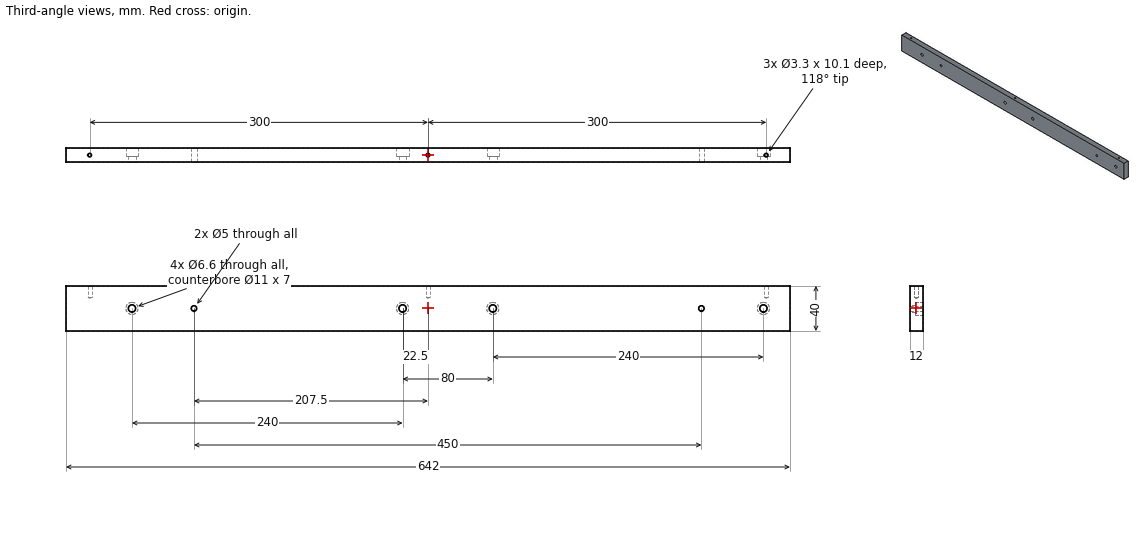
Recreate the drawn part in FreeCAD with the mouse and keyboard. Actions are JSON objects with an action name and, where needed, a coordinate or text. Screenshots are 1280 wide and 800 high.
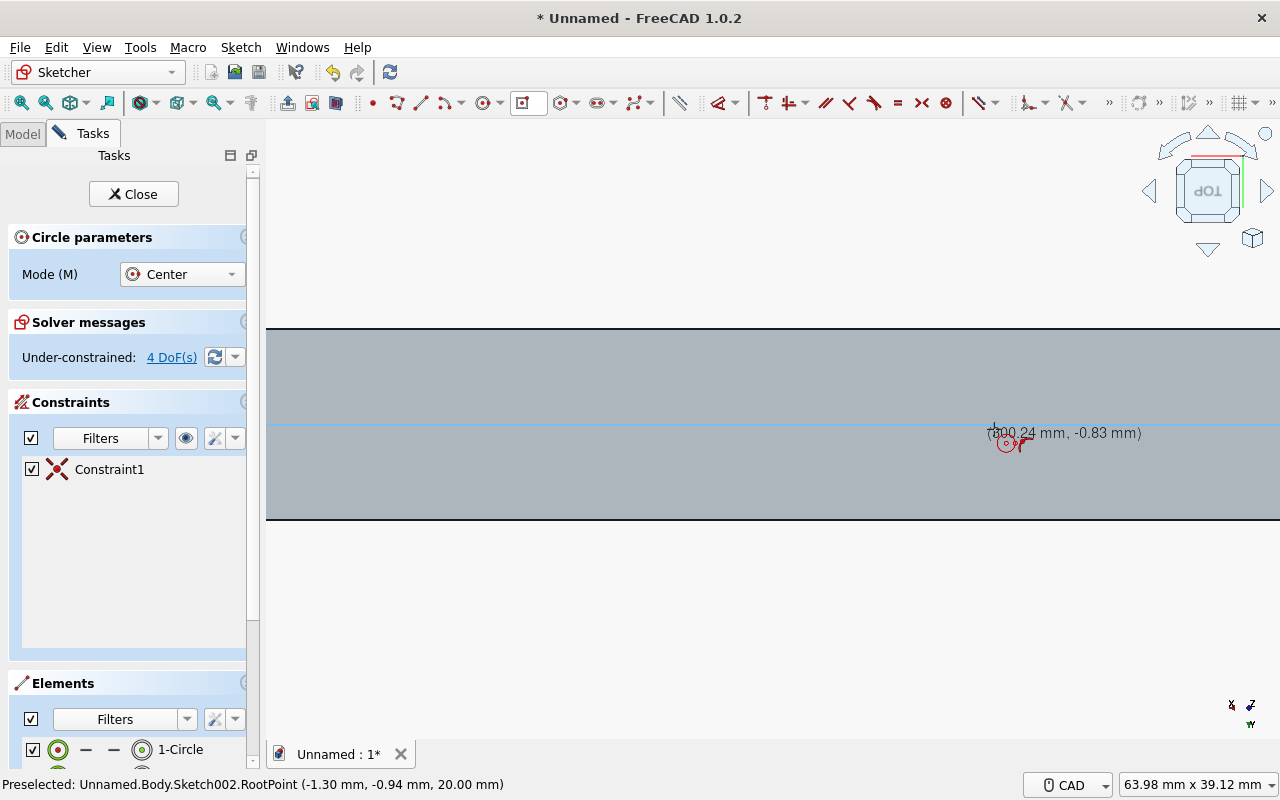
{"action": "scroll", "coordinate": [995, 429], "scroll_direction": "down", "scroll_amount": 14}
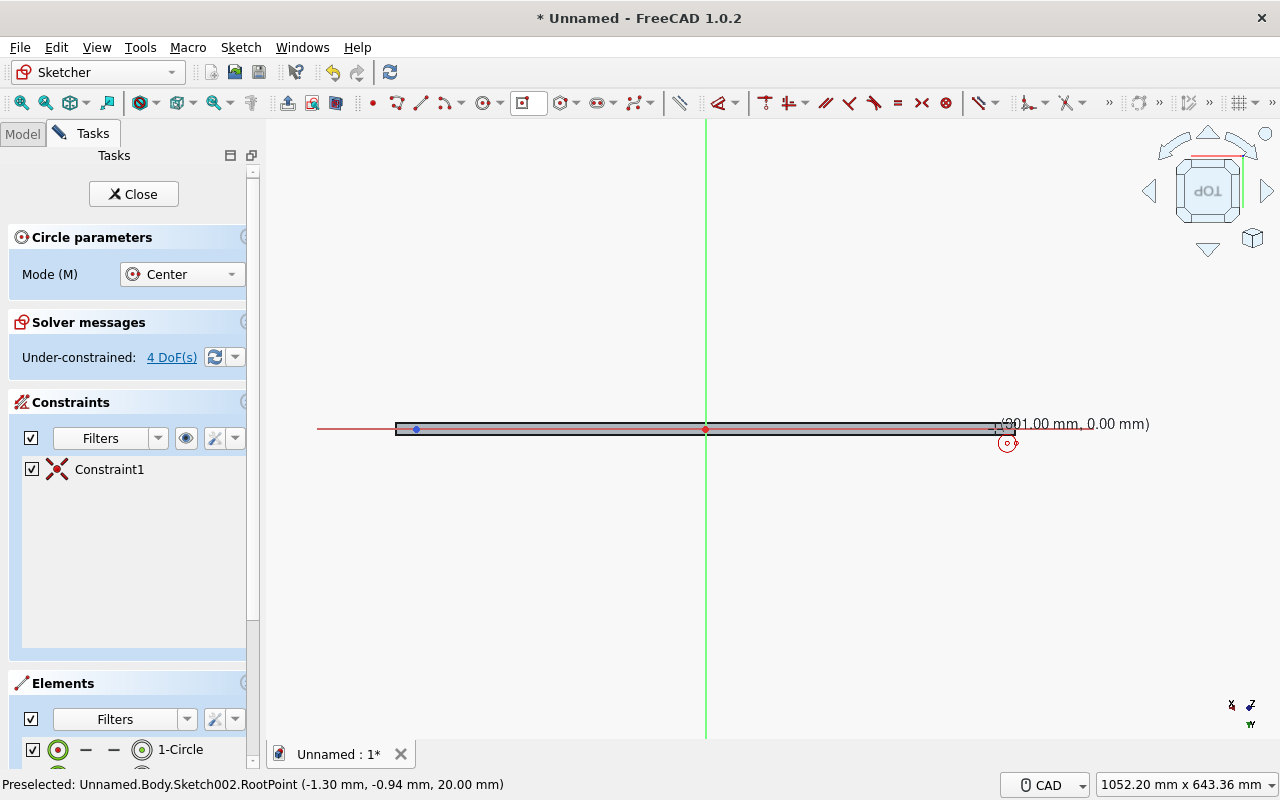
{"action": "left_click", "coordinate": [995, 429]}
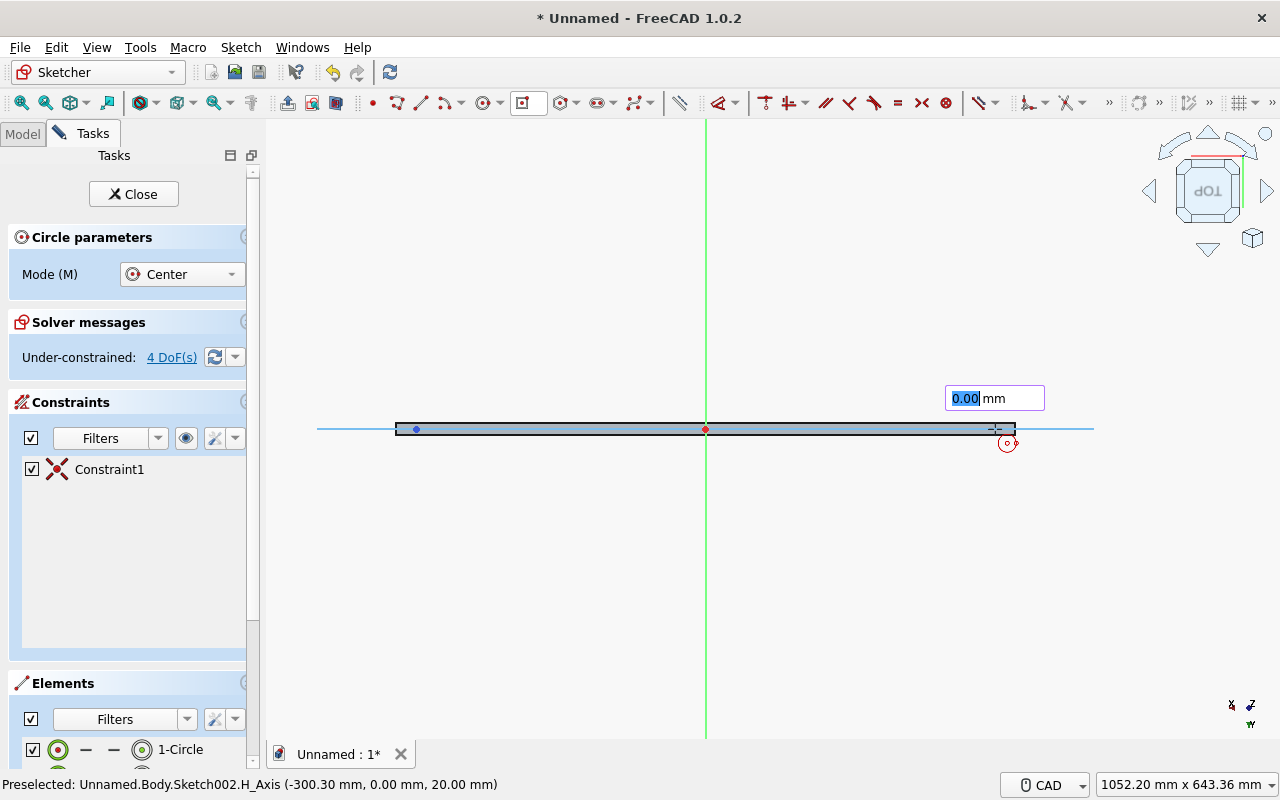
{"action": "scroll", "coordinate": [994, 431], "scroll_direction": "up", "scroll_amount": 12}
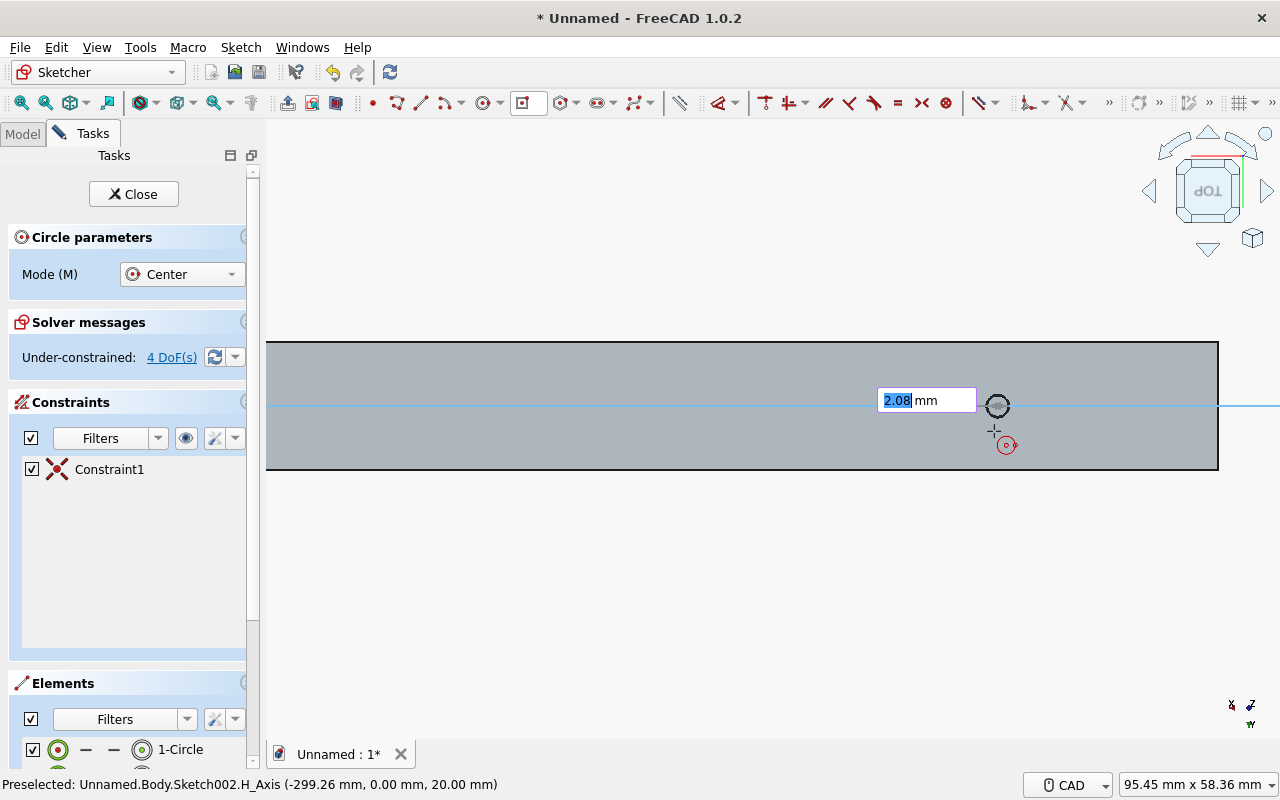
{"action": "left_click", "coordinate": [989, 423]}
{"action": "key", "text": "Escape"}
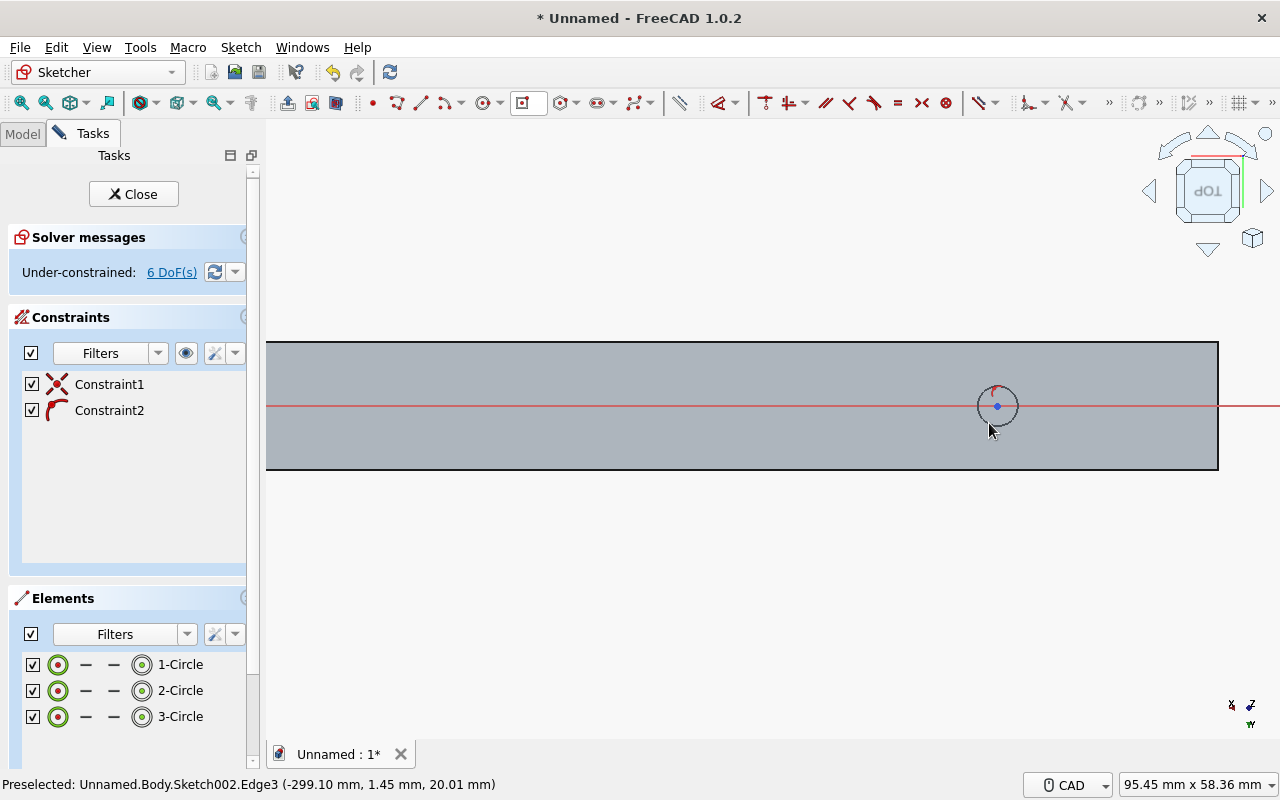
{"action": "scroll", "coordinate": [994, 431], "scroll_direction": "down", "scroll_amount": 12}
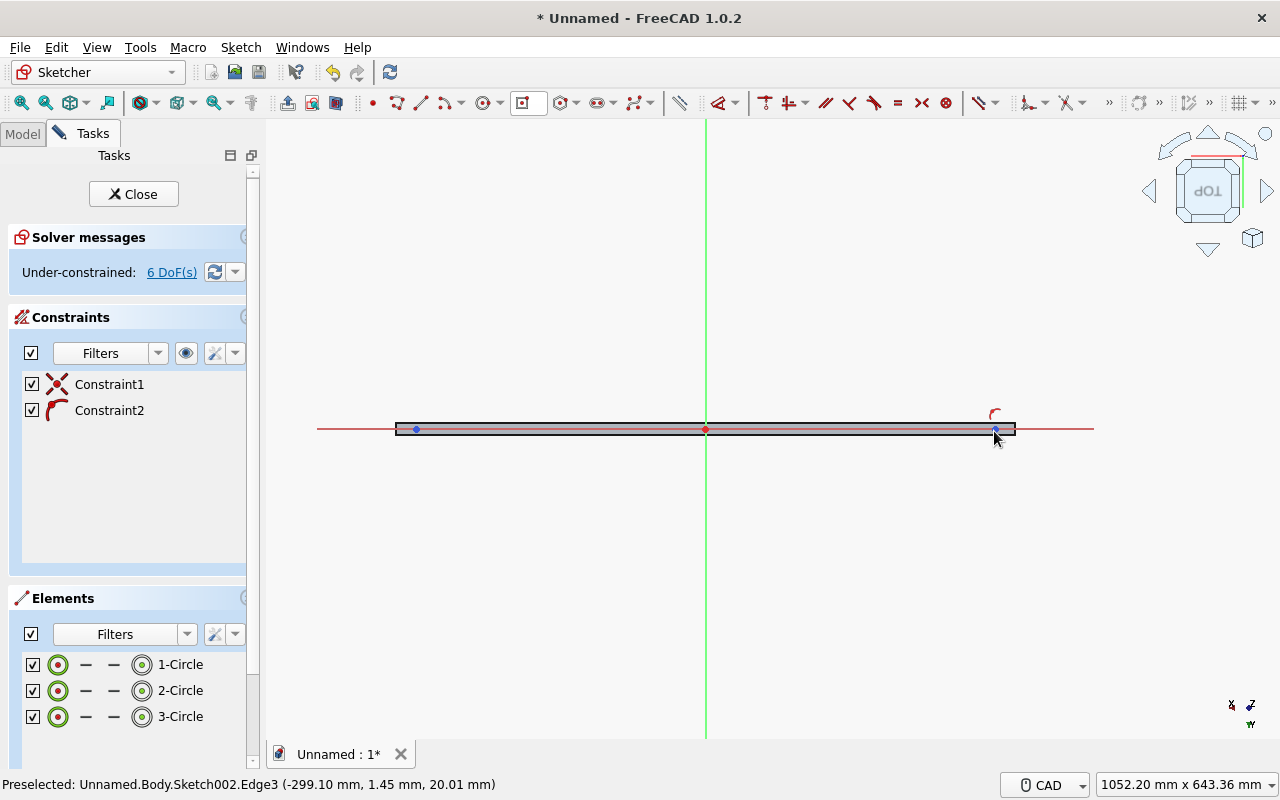
{"action": "scroll", "coordinate": [418, 429], "scroll_direction": "up", "scroll_amount": 12}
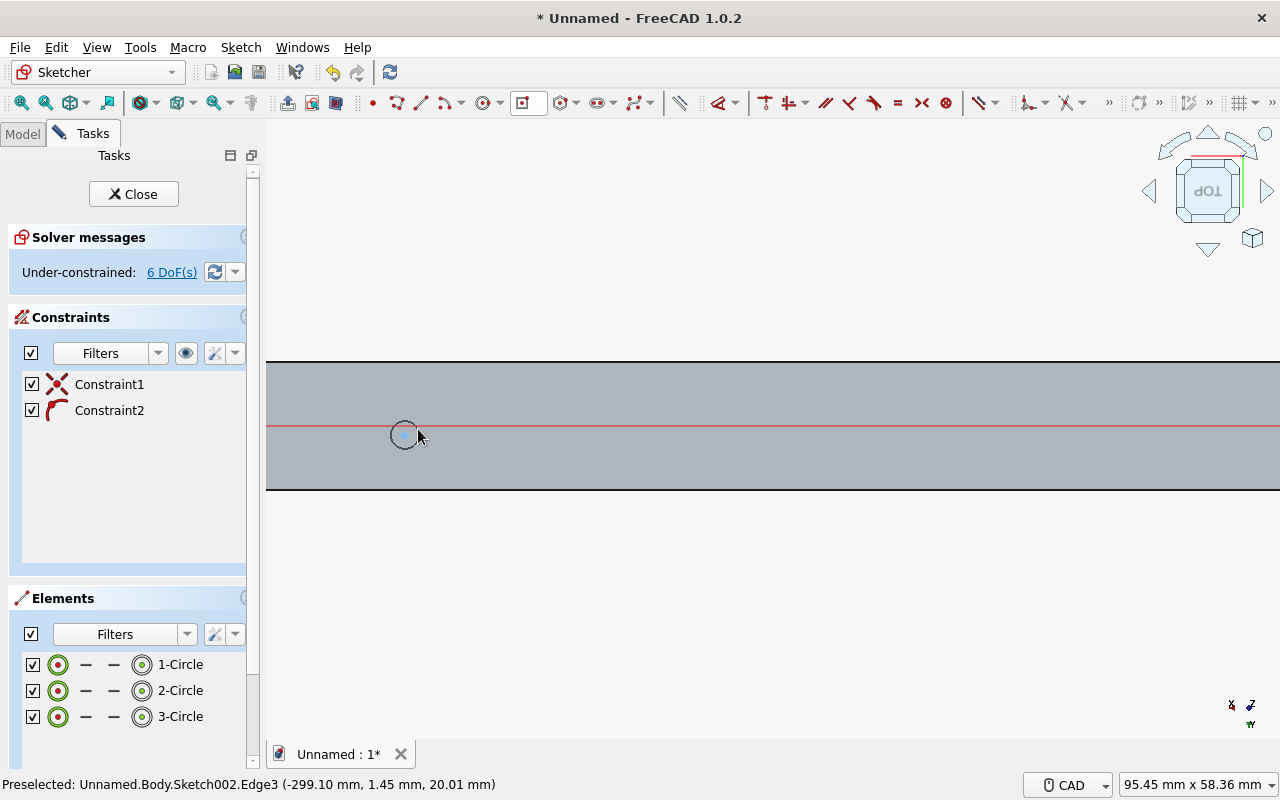
{"action": "left_click", "coordinate": [415, 425]}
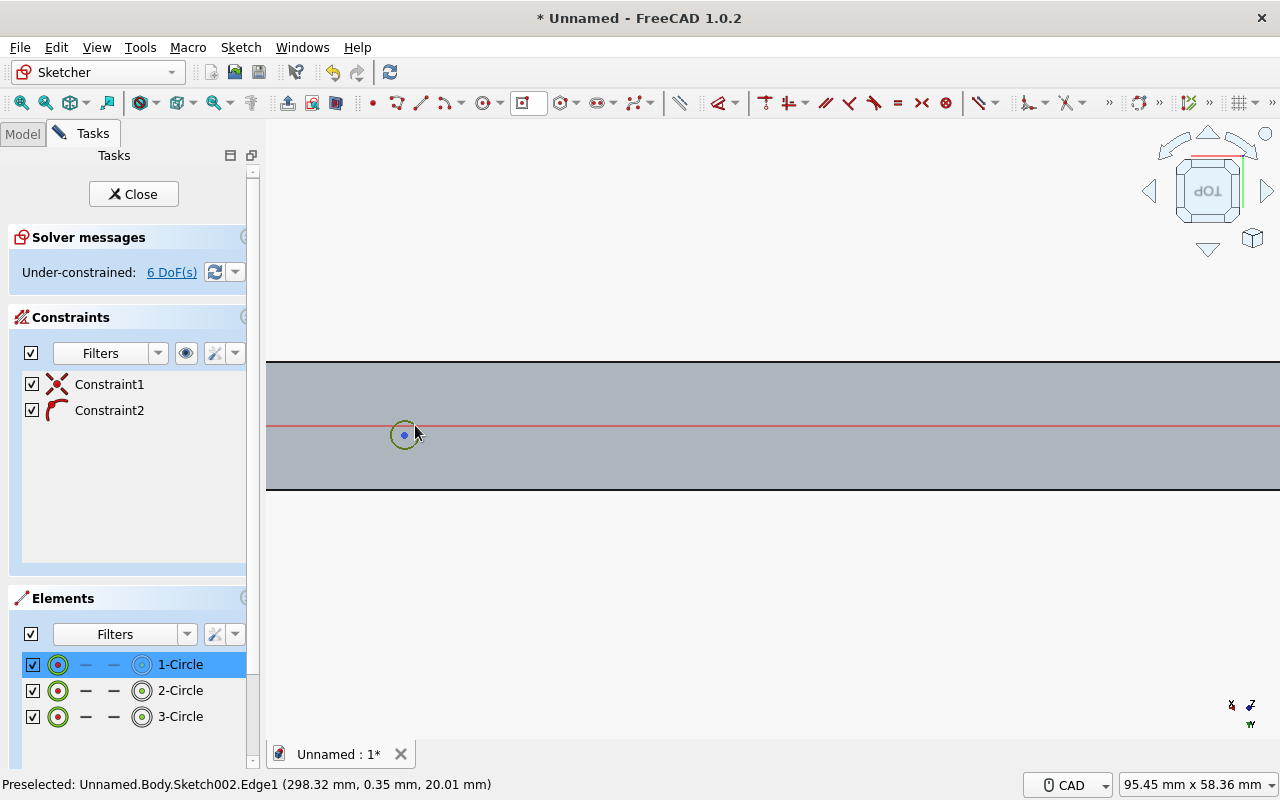
{"action": "scroll", "coordinate": [417, 429], "scroll_direction": "down", "scroll_amount": 12}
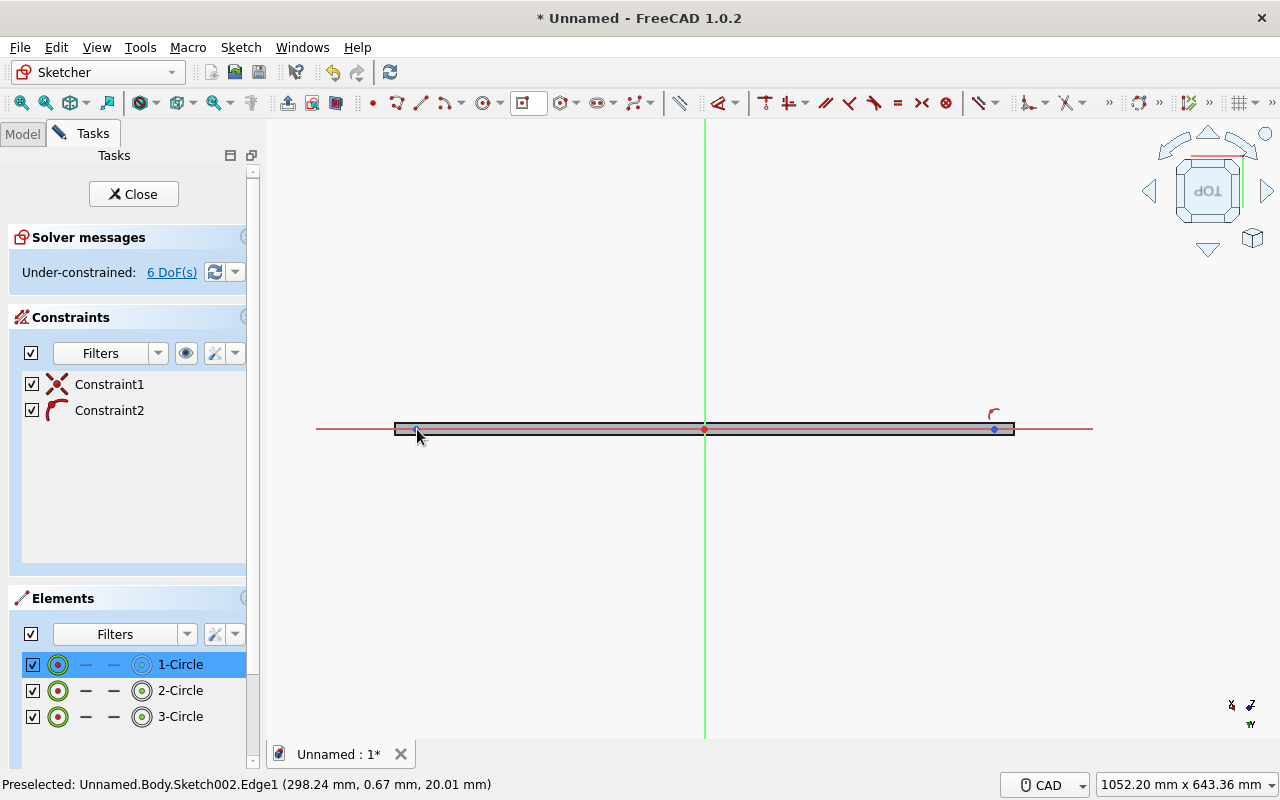
{"action": "scroll", "coordinate": [706, 428], "scroll_direction": "up", "scroll_amount": 13}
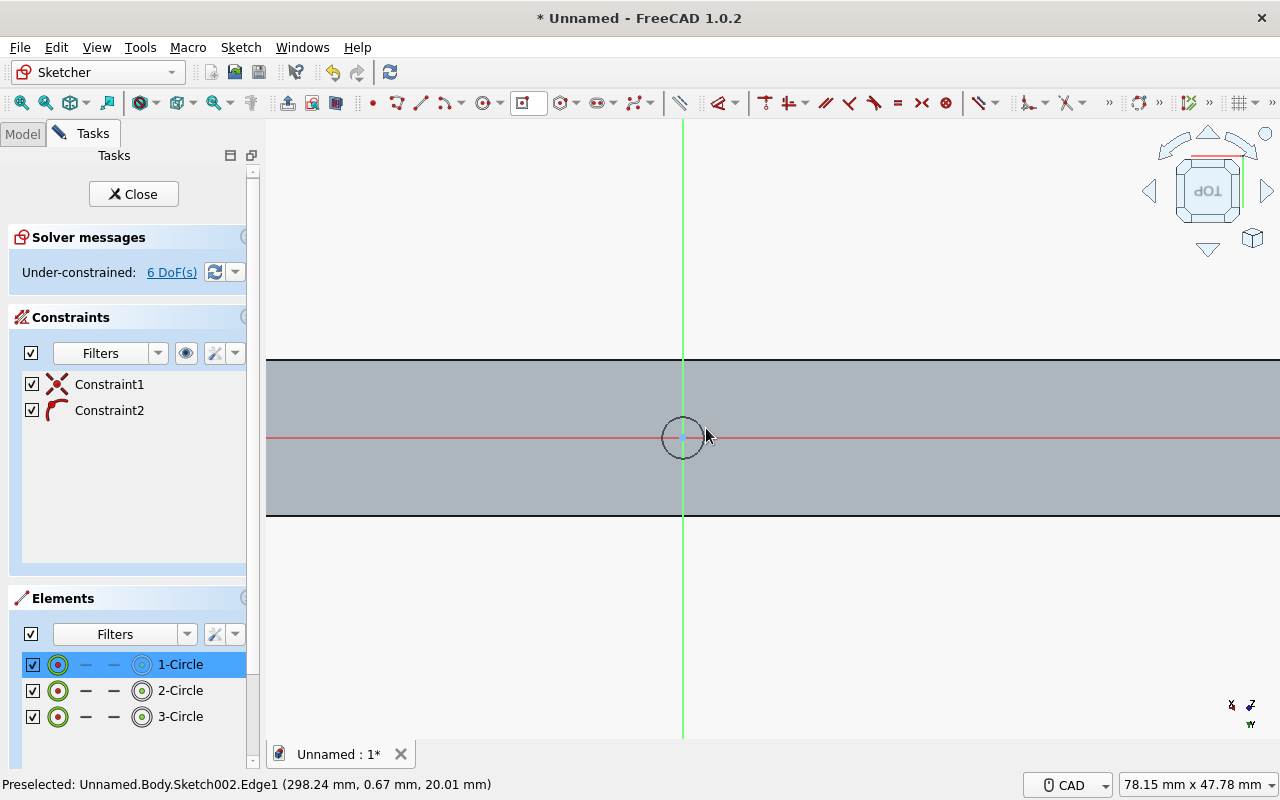
{"action": "left_click", "coordinate": [698, 423]}